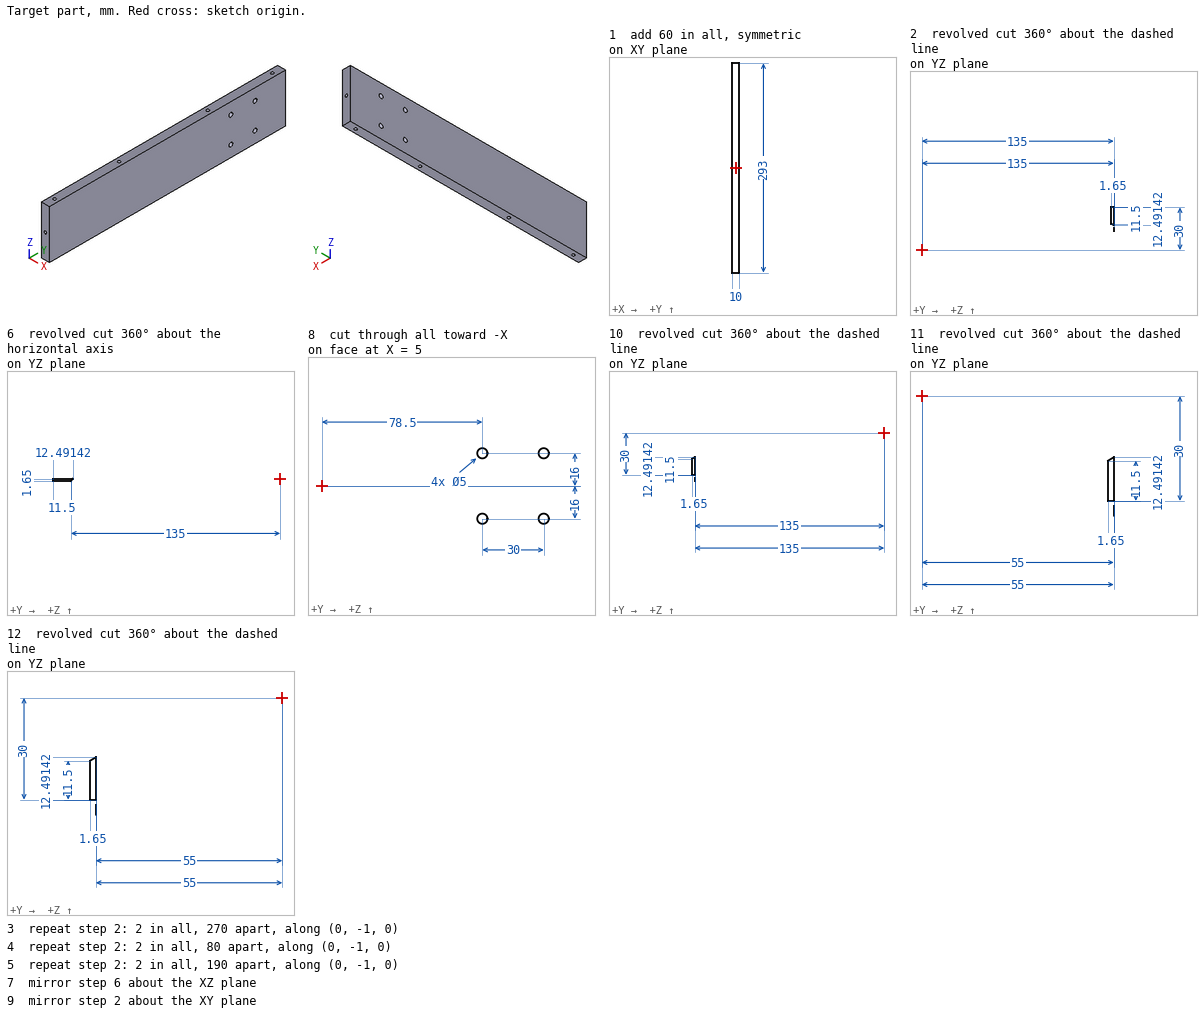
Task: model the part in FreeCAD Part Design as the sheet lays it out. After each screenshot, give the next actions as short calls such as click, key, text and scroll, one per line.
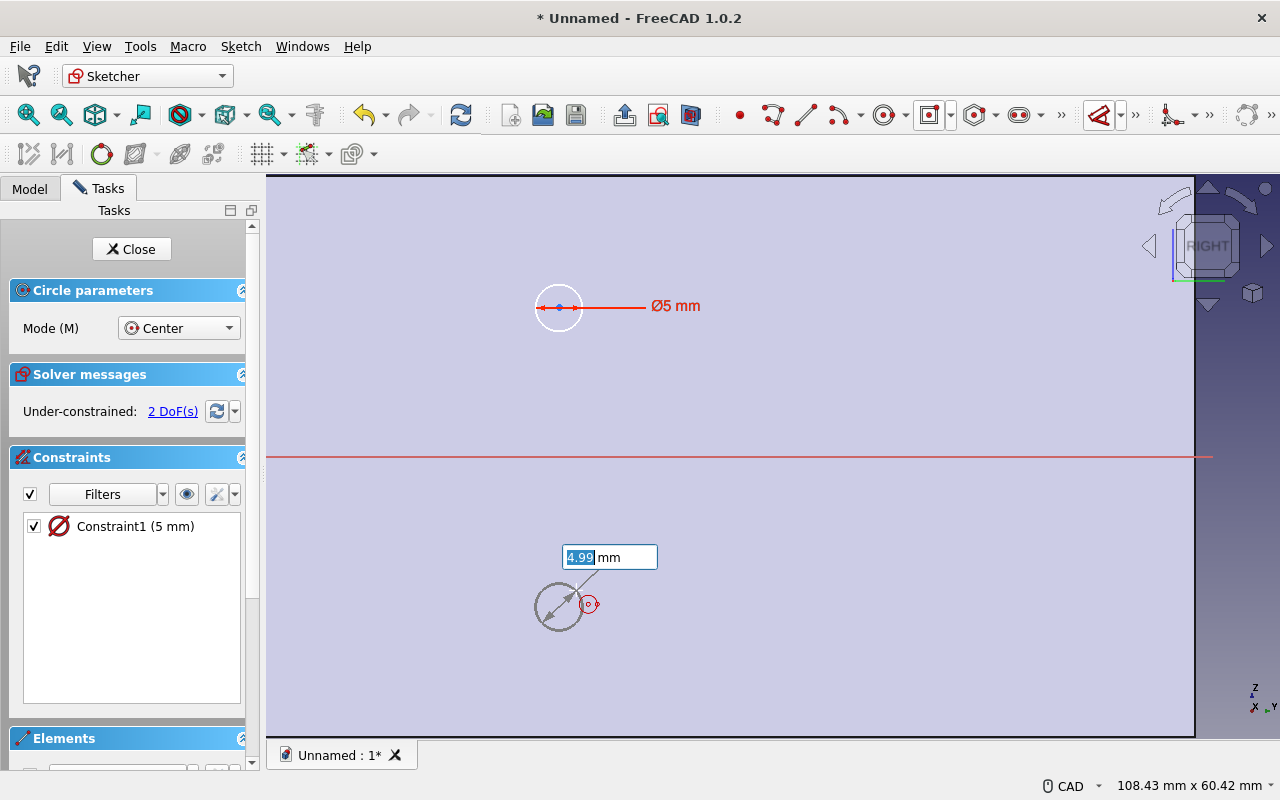
text(5)
key(Return)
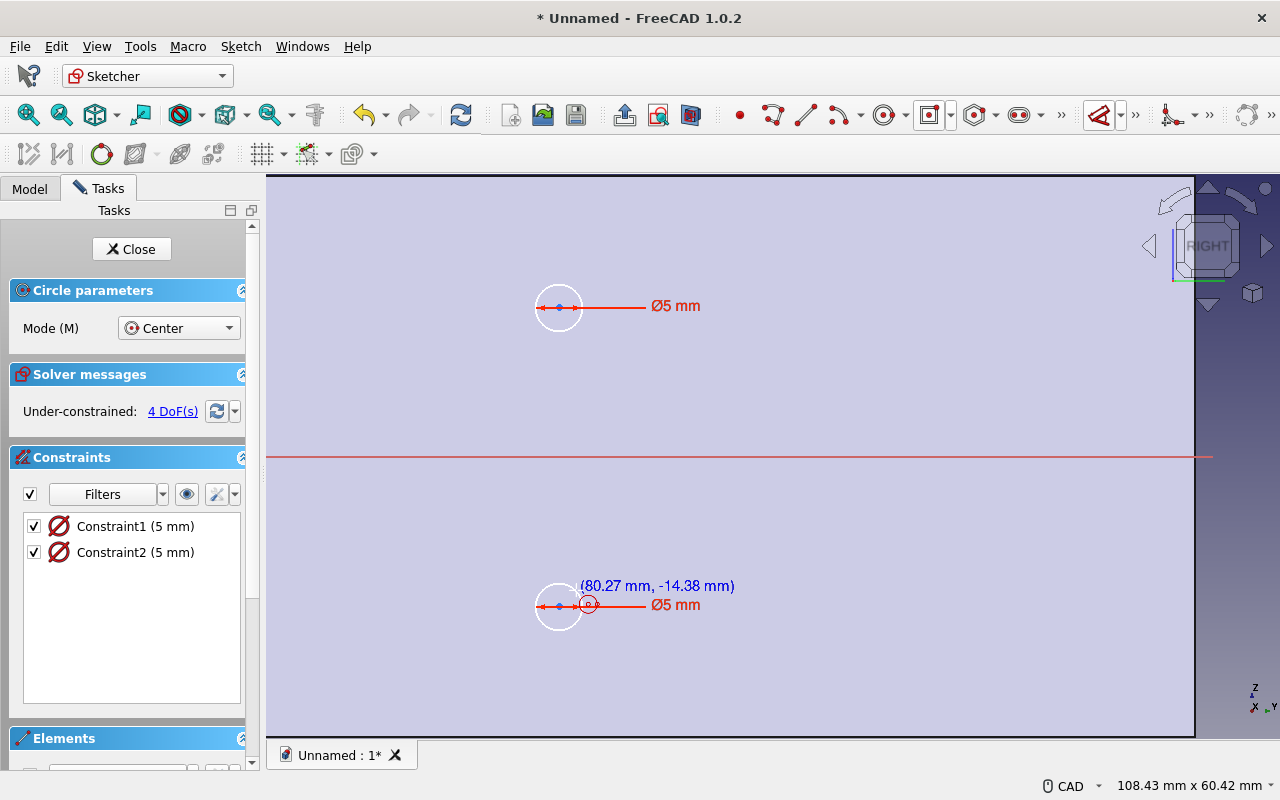
click(840, 606)
move(857, 590)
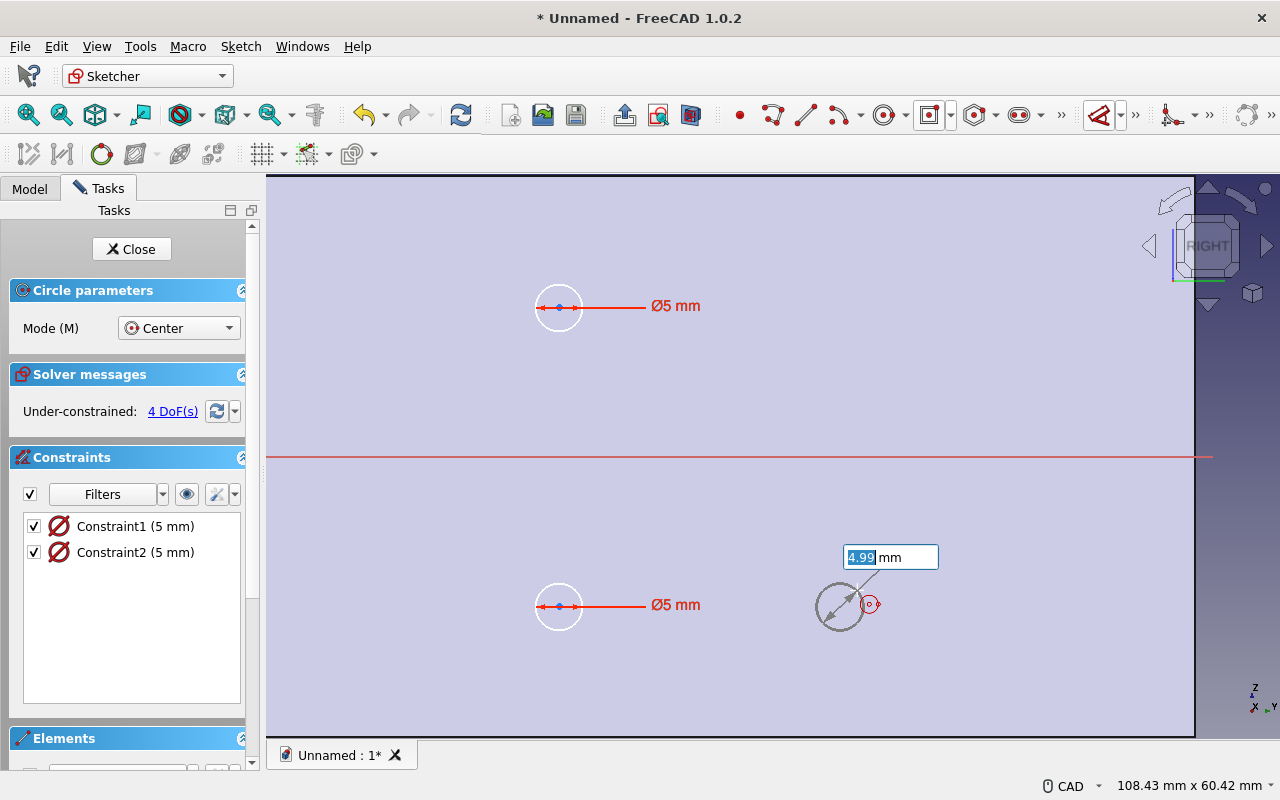
text(5)
key(Return)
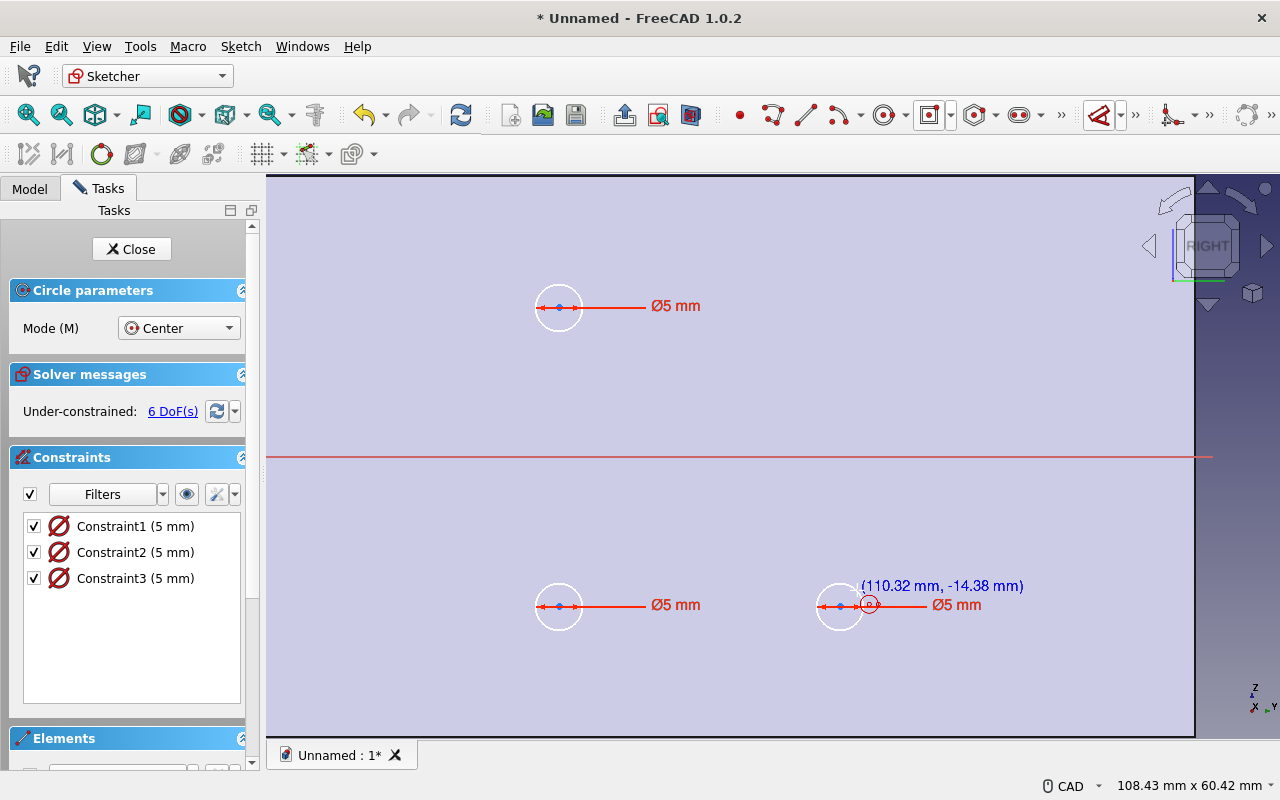
click(840, 307)
move(857, 290)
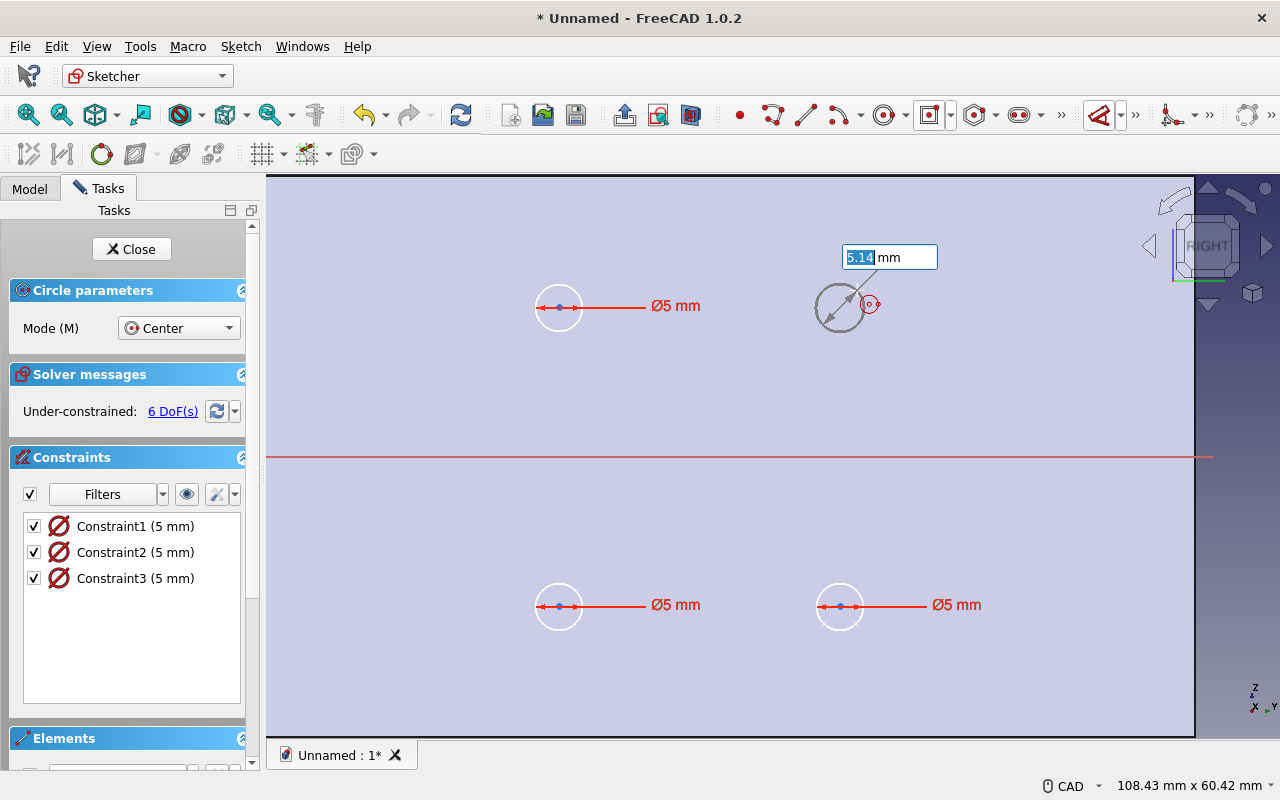
text(5)
key(Return)
key(Escape)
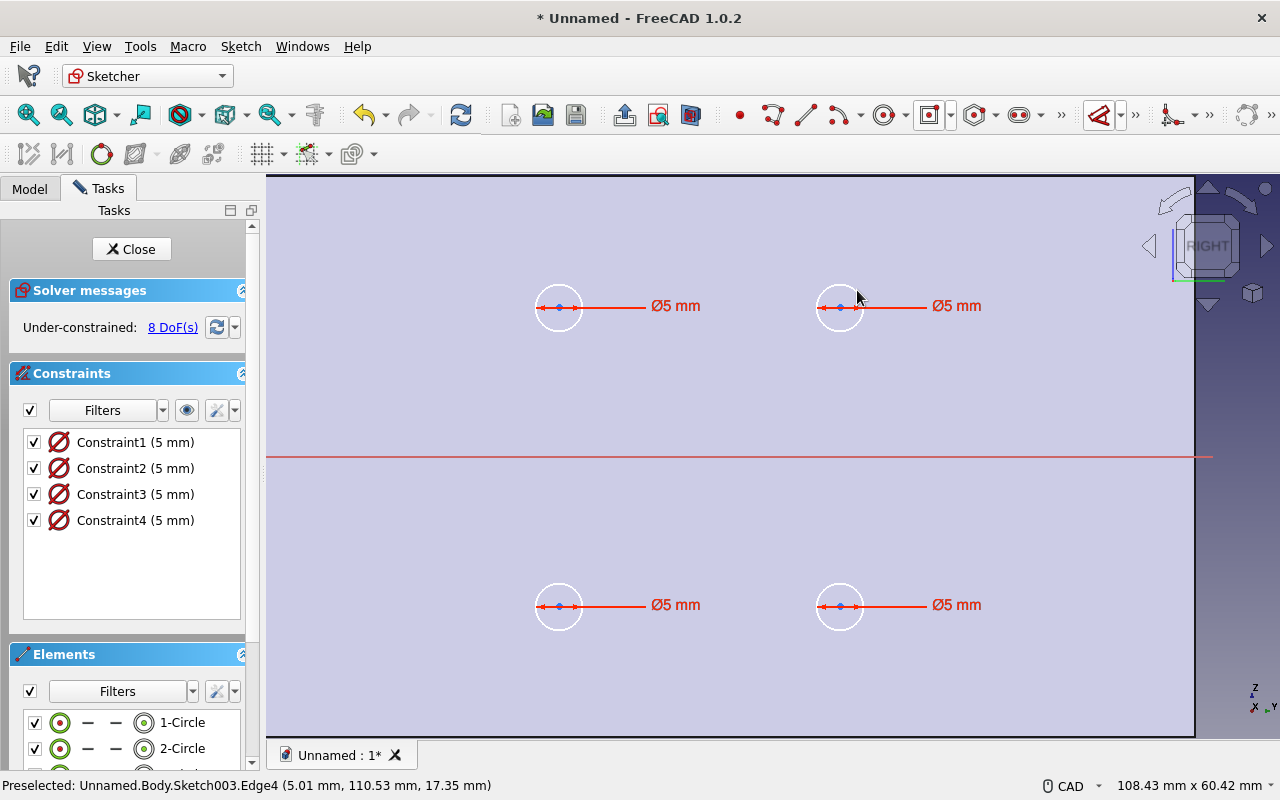
click(559, 308)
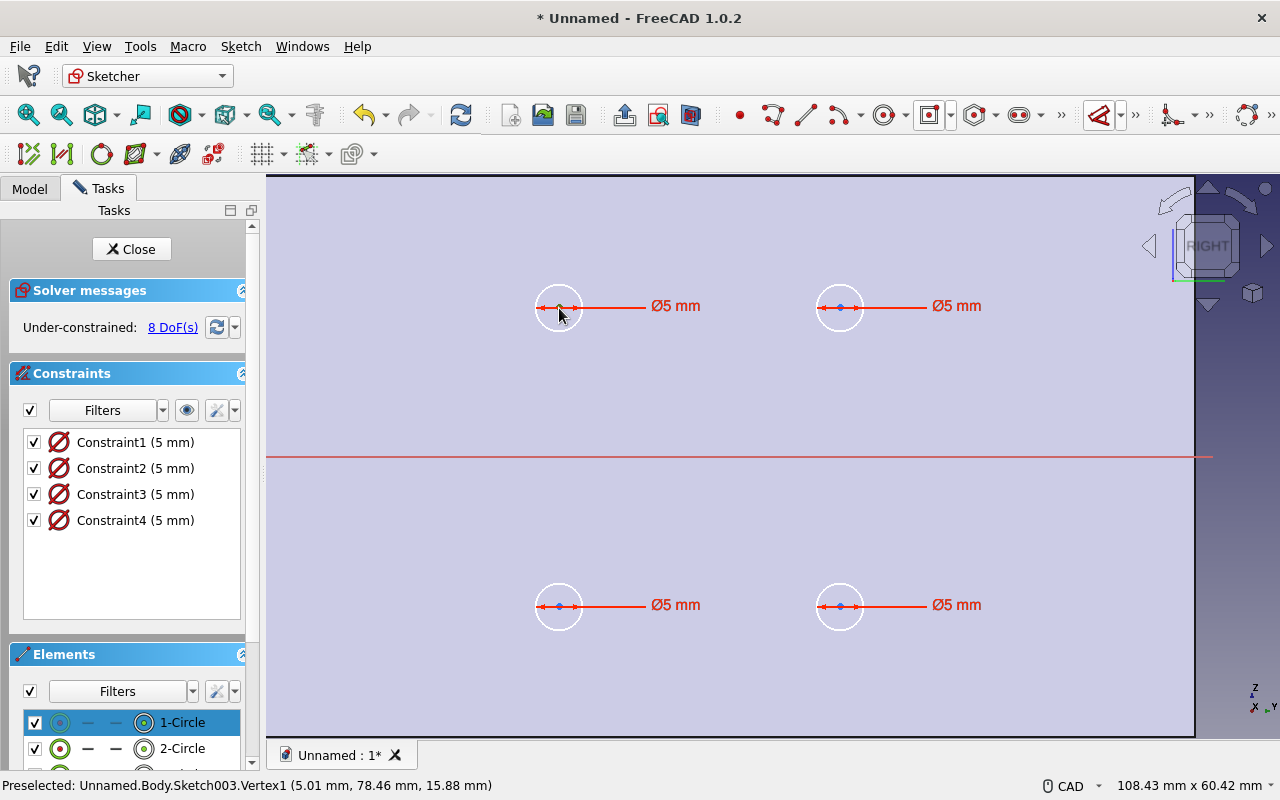
click(559, 607)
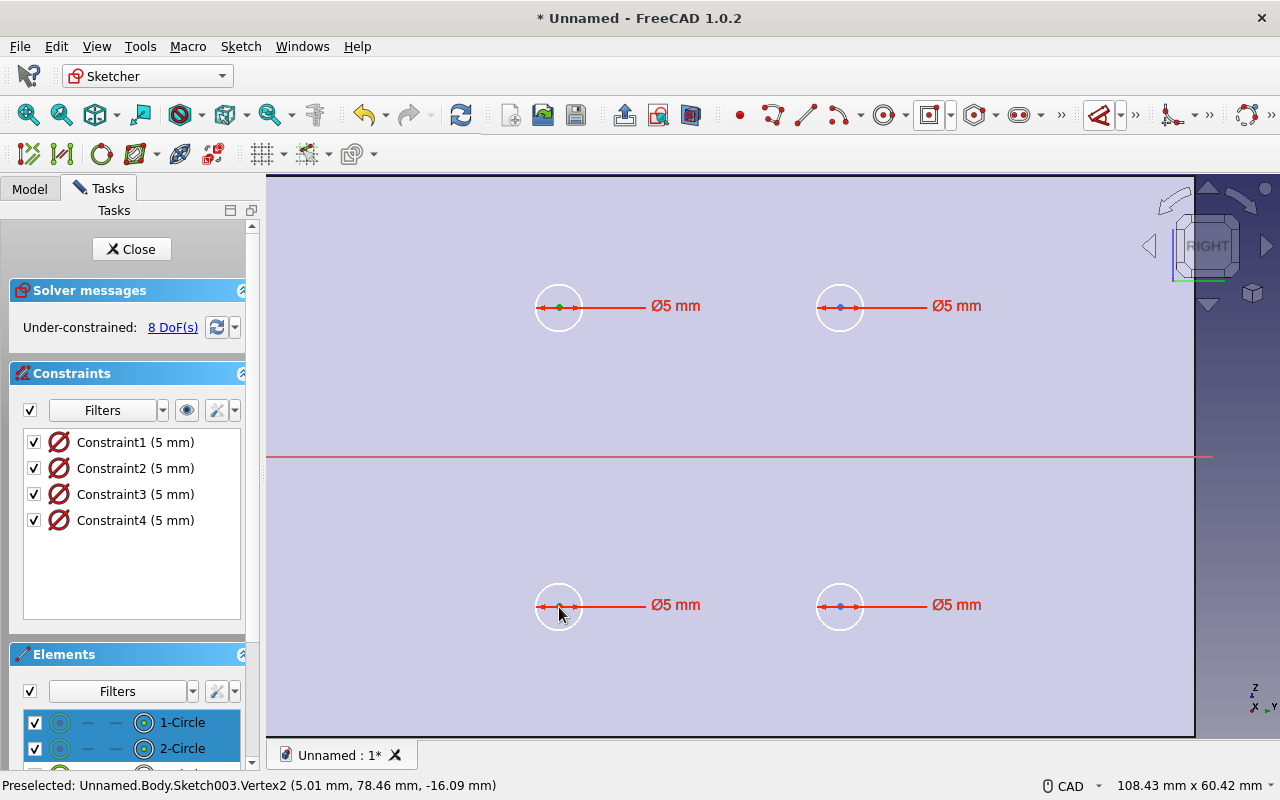
key(v)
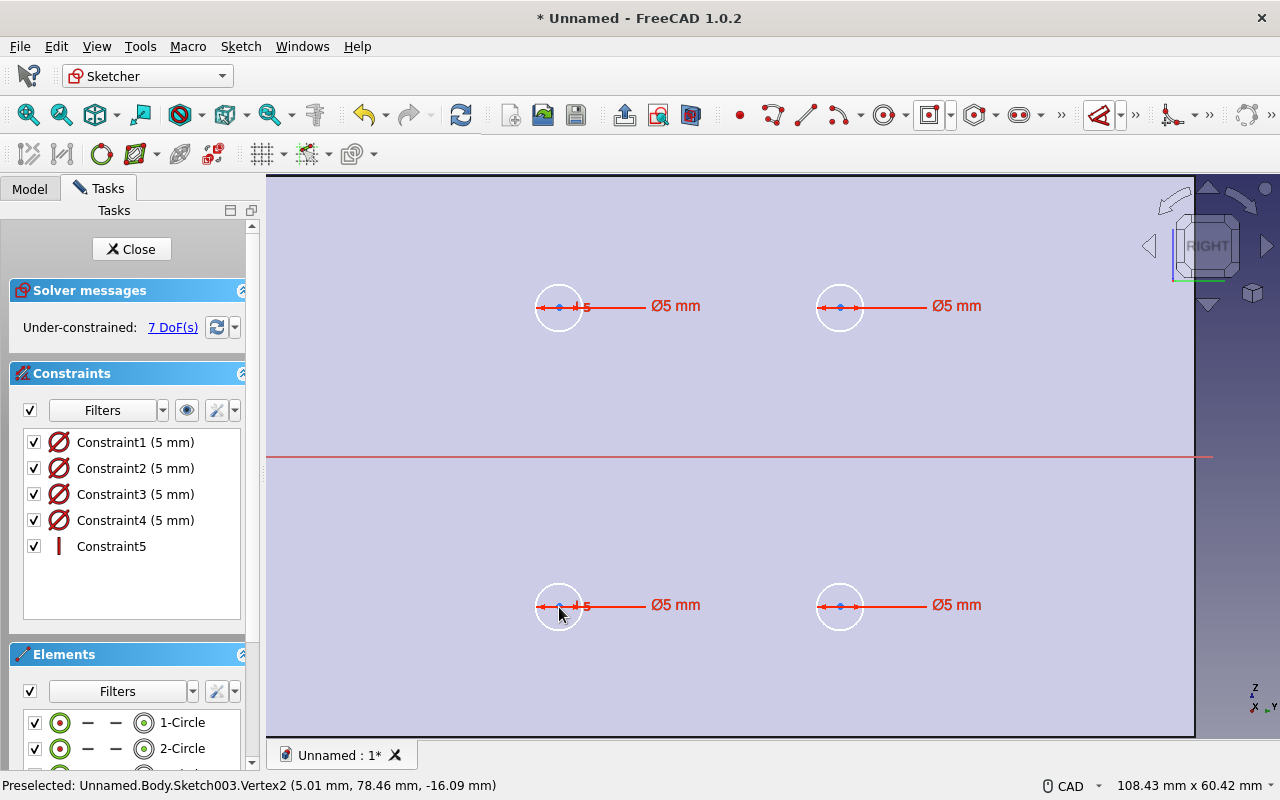
click(559, 607)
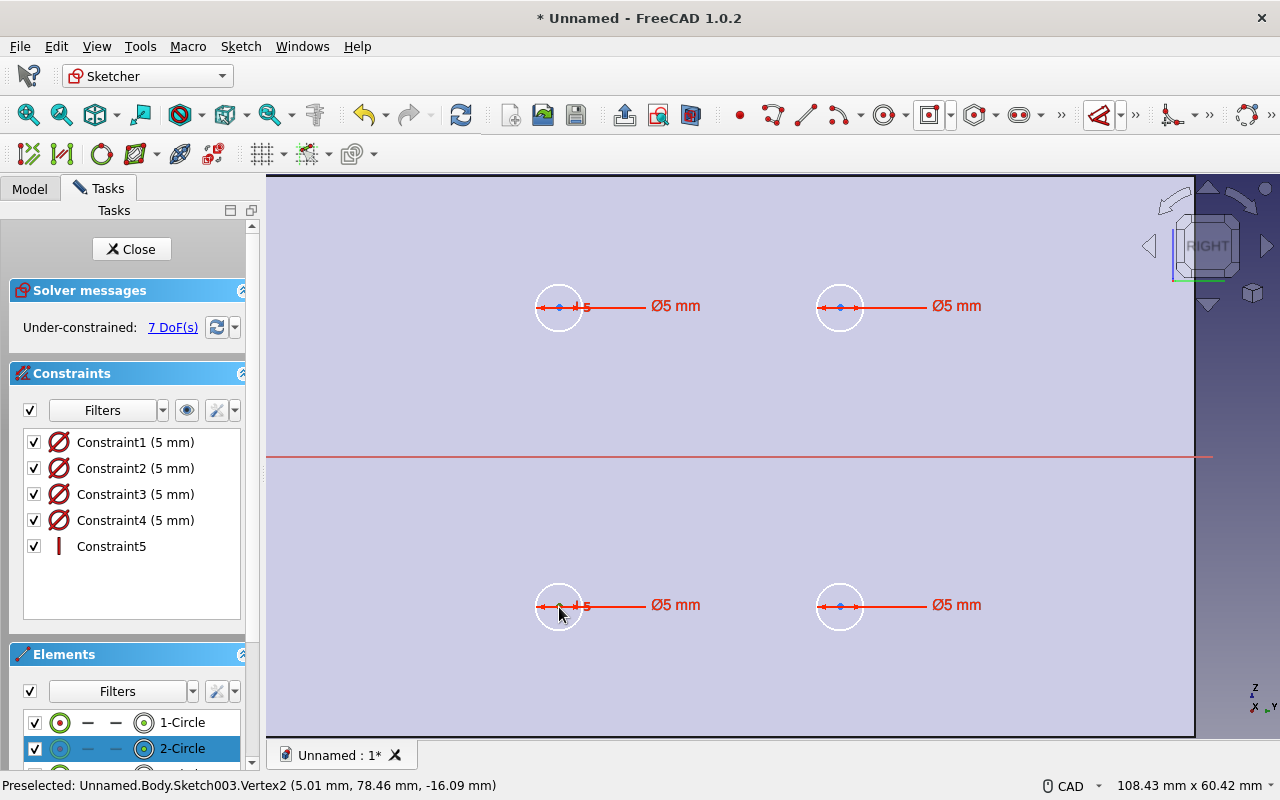
click(840, 607)